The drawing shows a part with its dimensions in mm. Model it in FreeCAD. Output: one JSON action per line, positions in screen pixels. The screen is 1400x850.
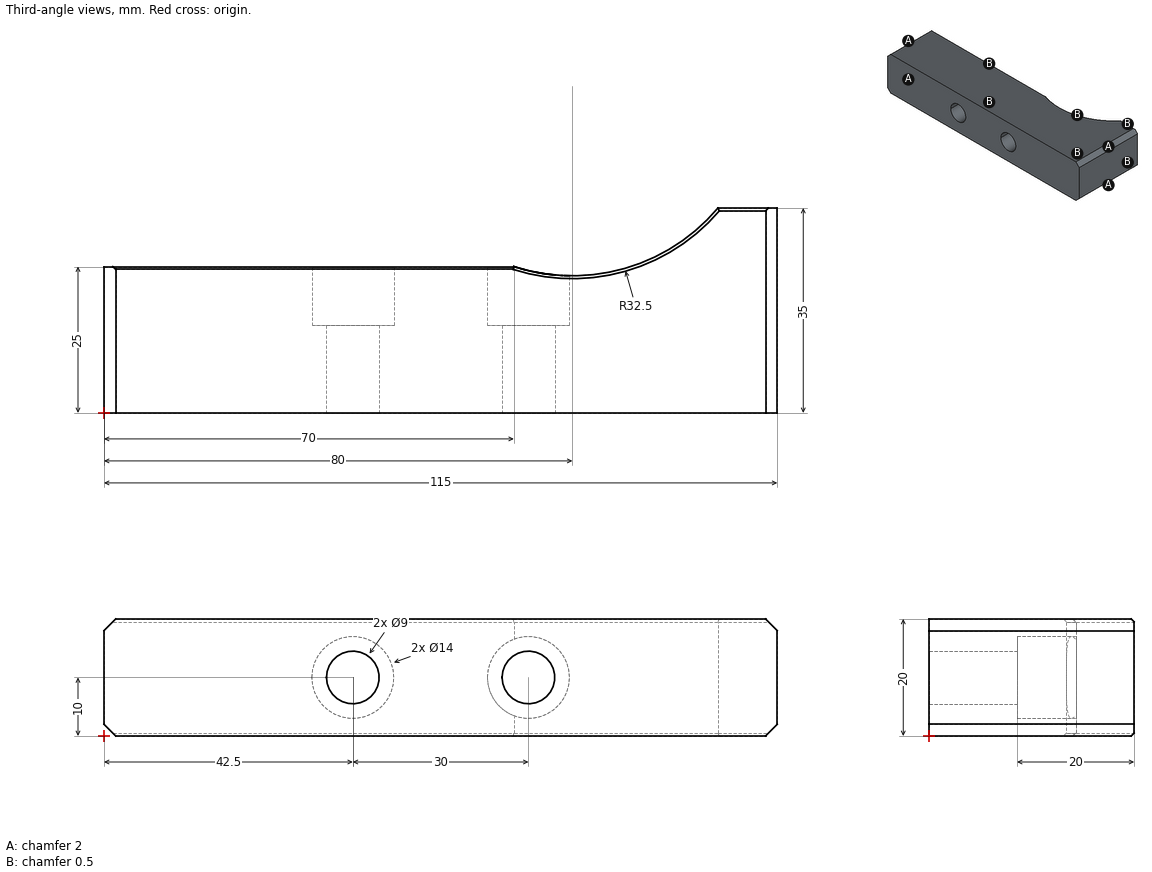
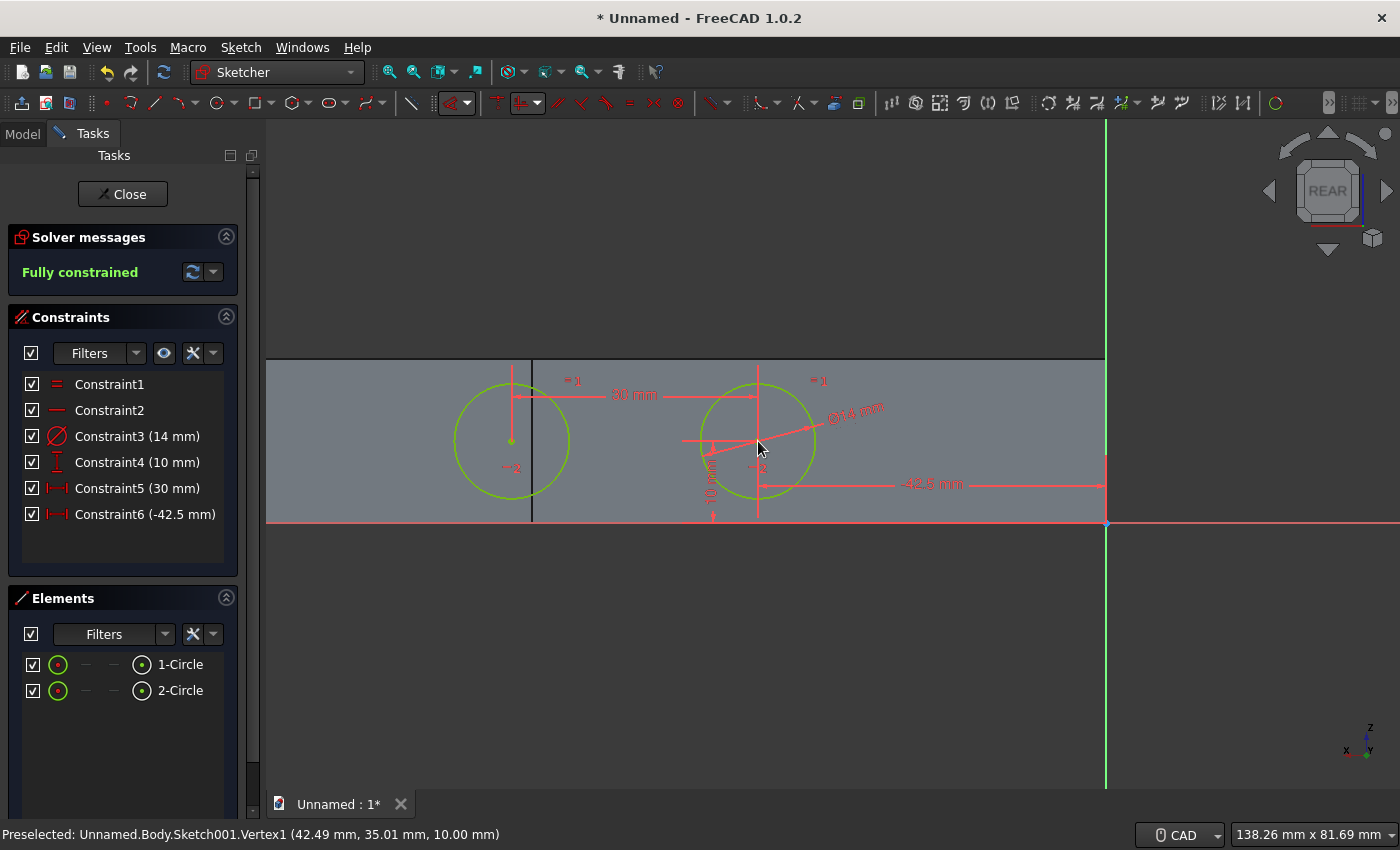
{"action": "left_click", "coordinate": [123, 194]}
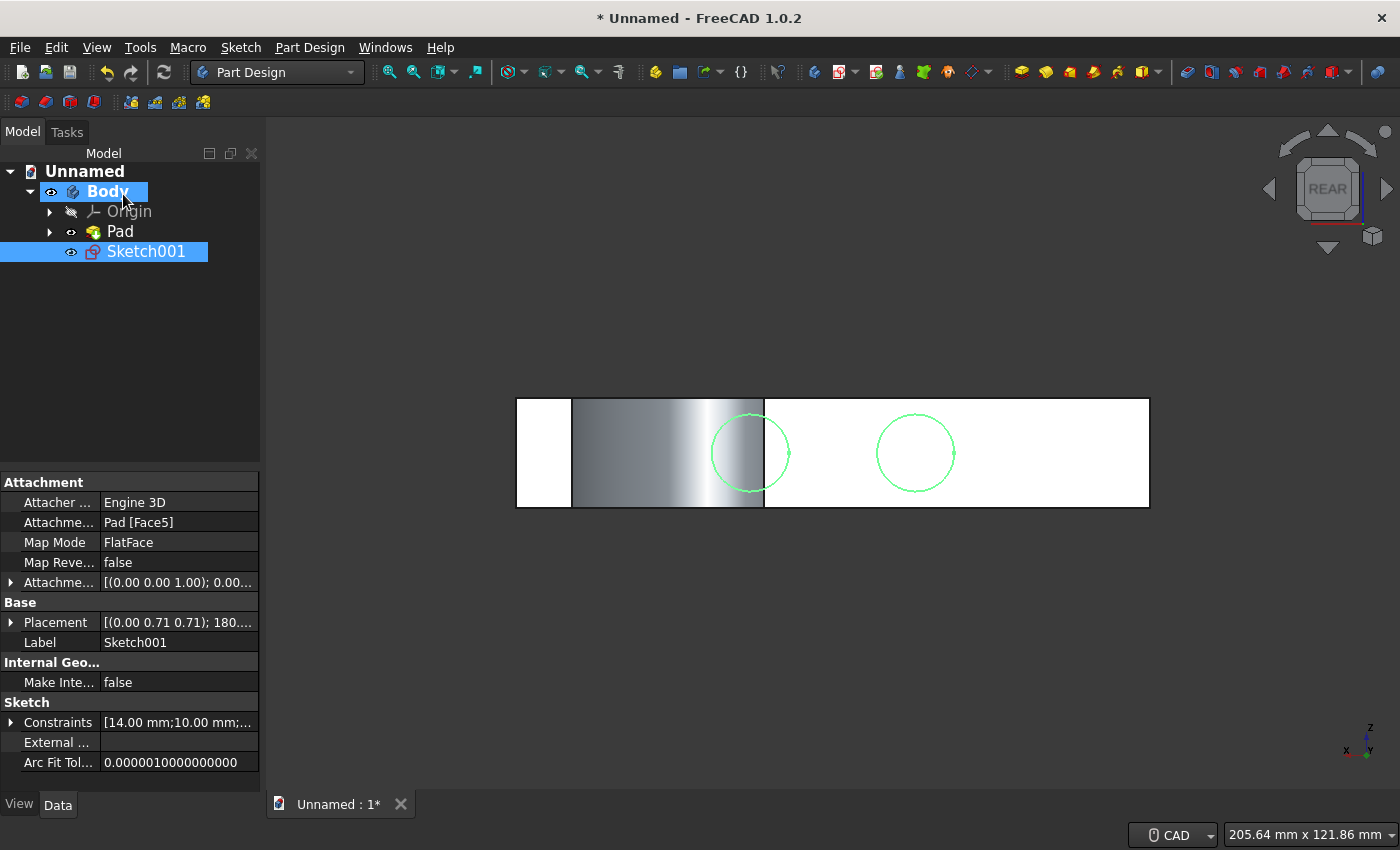
{"action": "left_click", "coordinate": [1188, 72]}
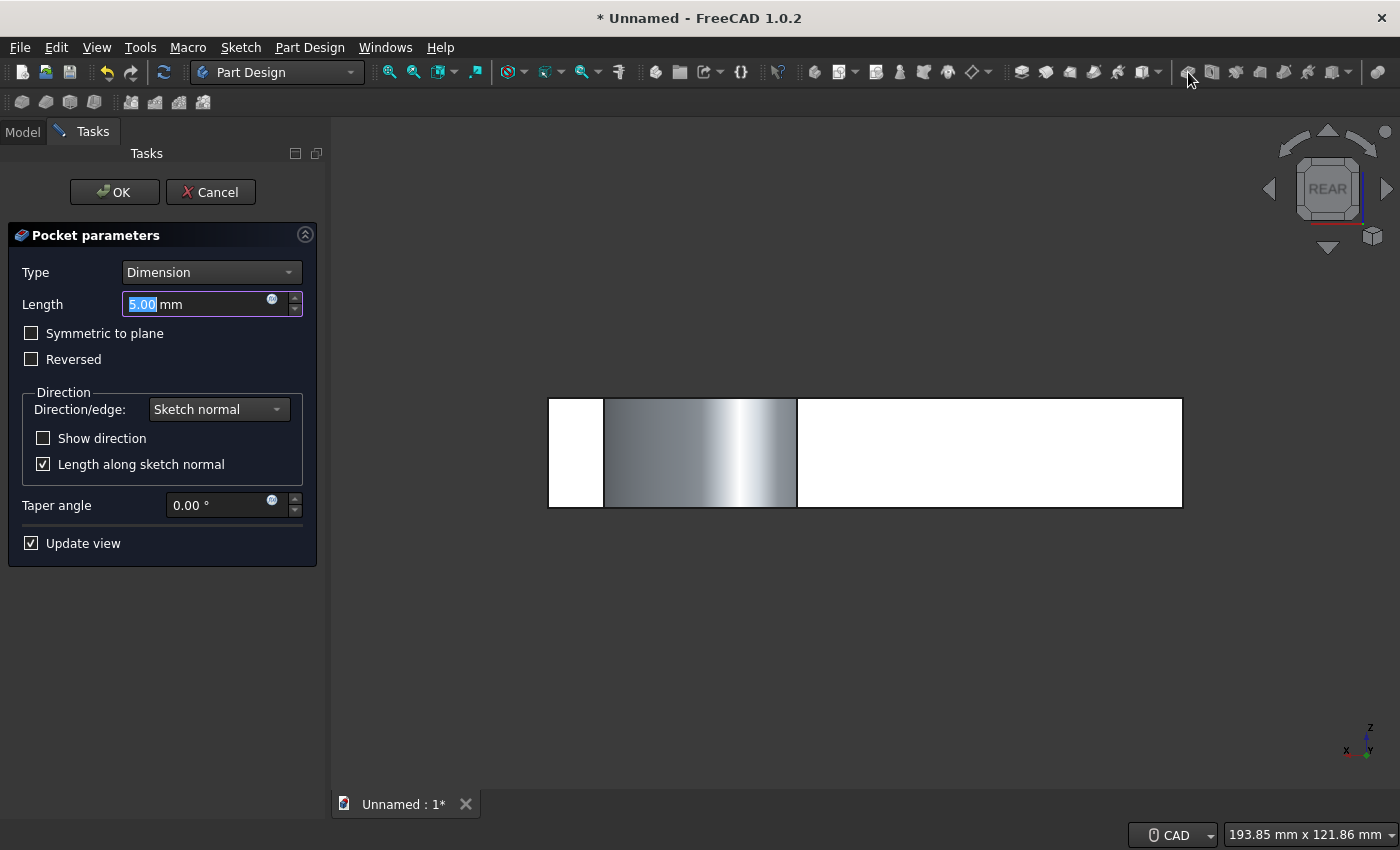
{"action": "type", "text": "20"}
{"action": "key", "text": "Tab"}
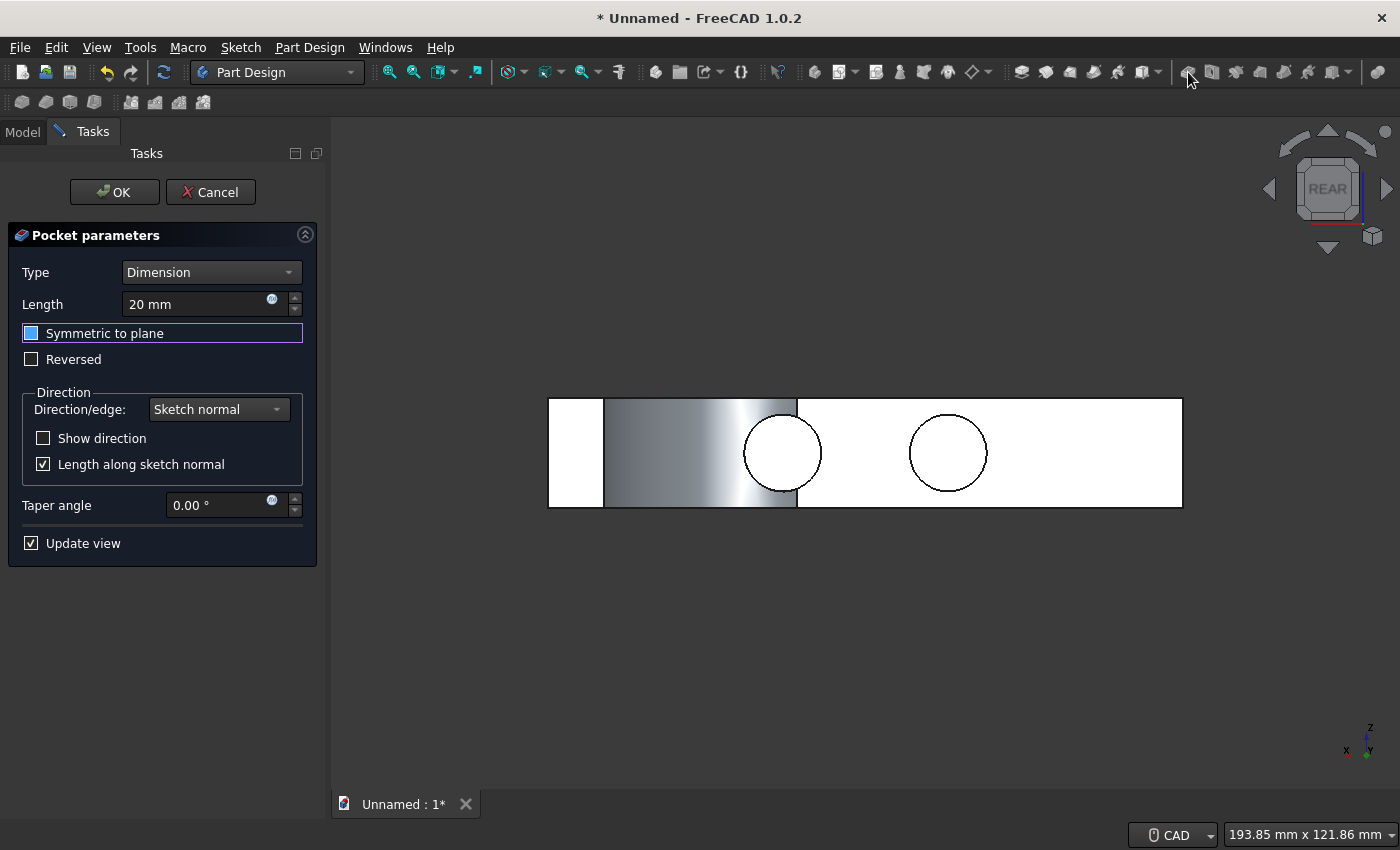
{"action": "left_click", "coordinate": [115, 192]}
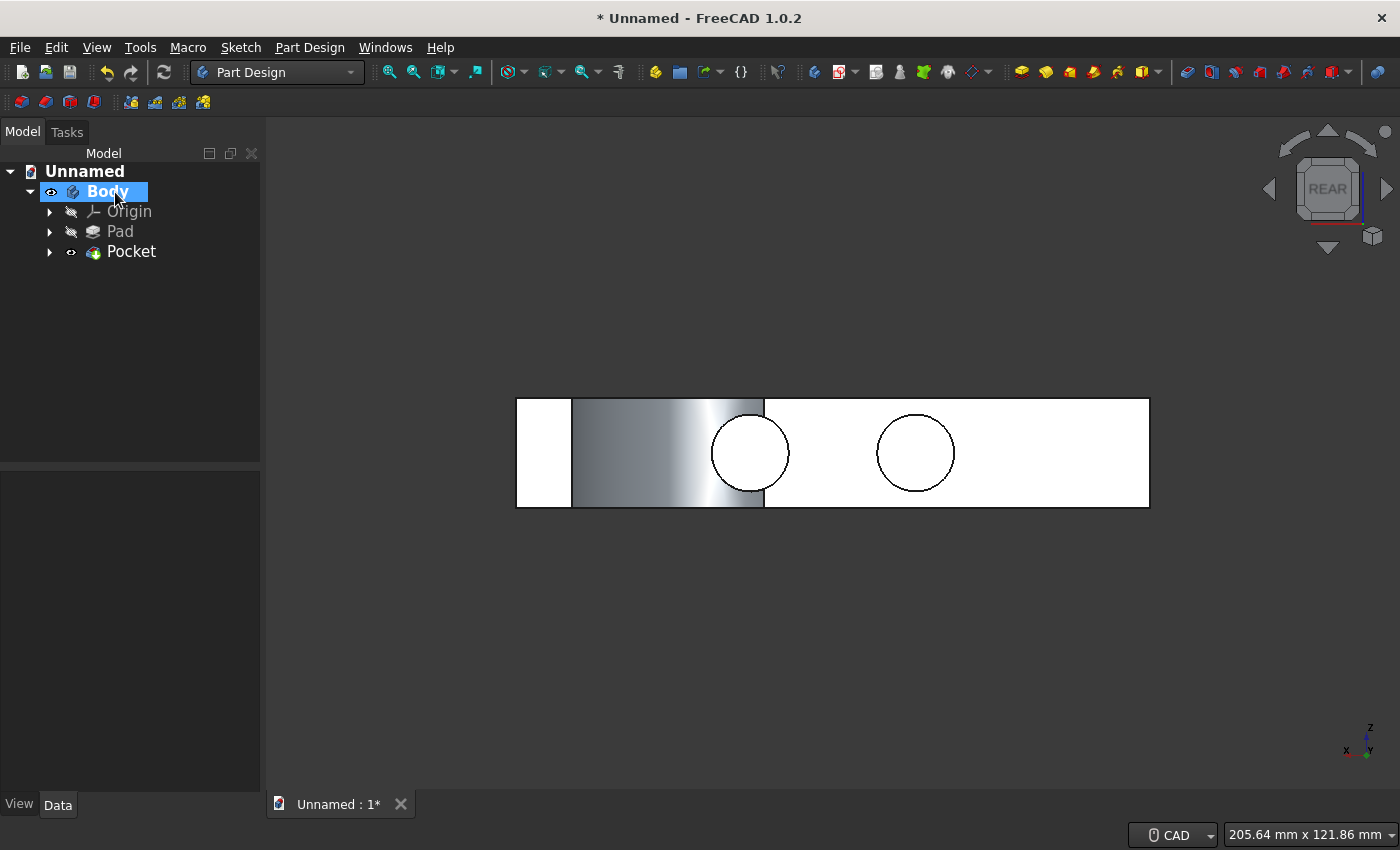
{"action": "left_click", "coordinate": [916, 452]}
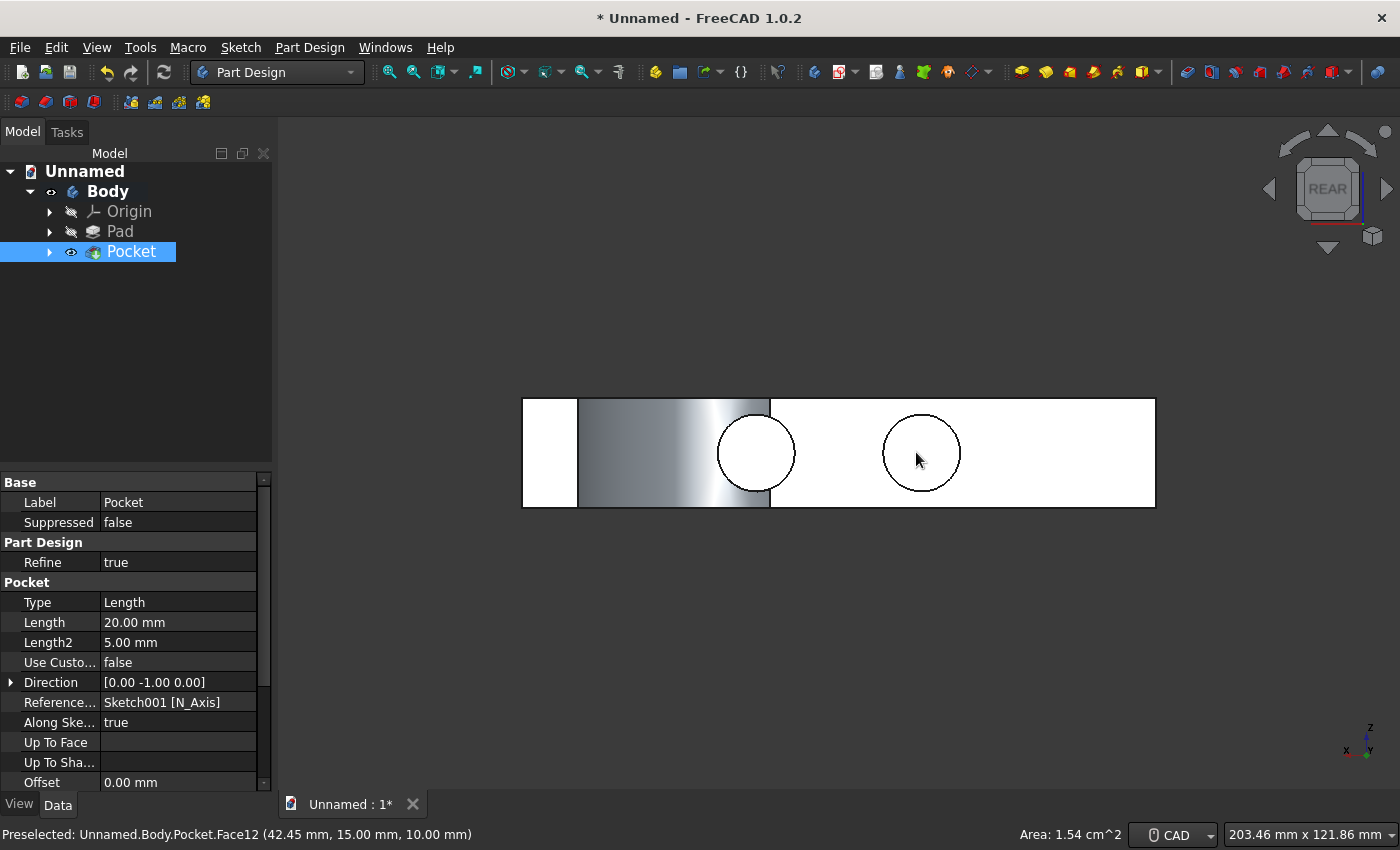
{"action": "left_click", "coordinate": [840, 72]}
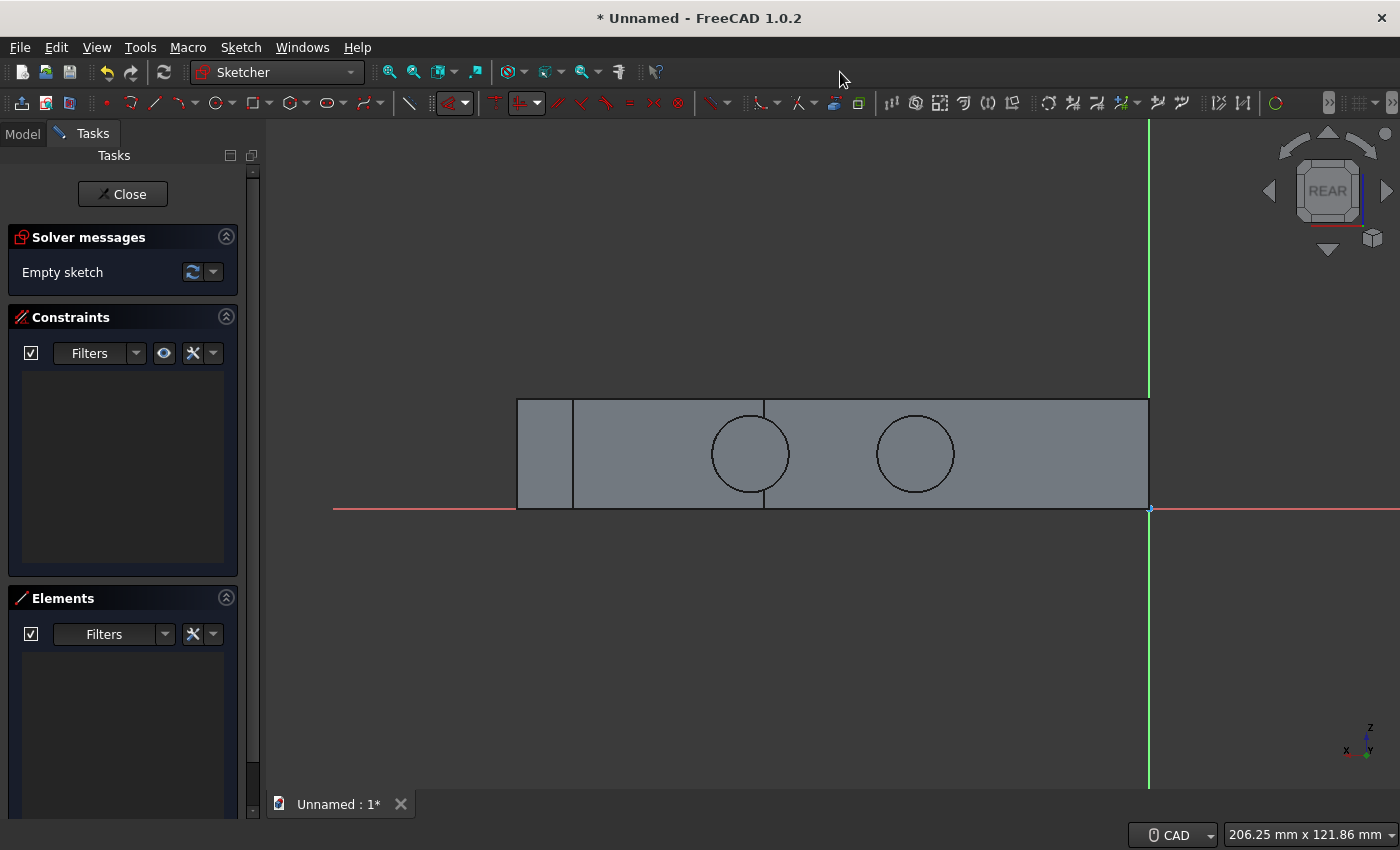
{"action": "left_click", "coordinate": [70, 104]}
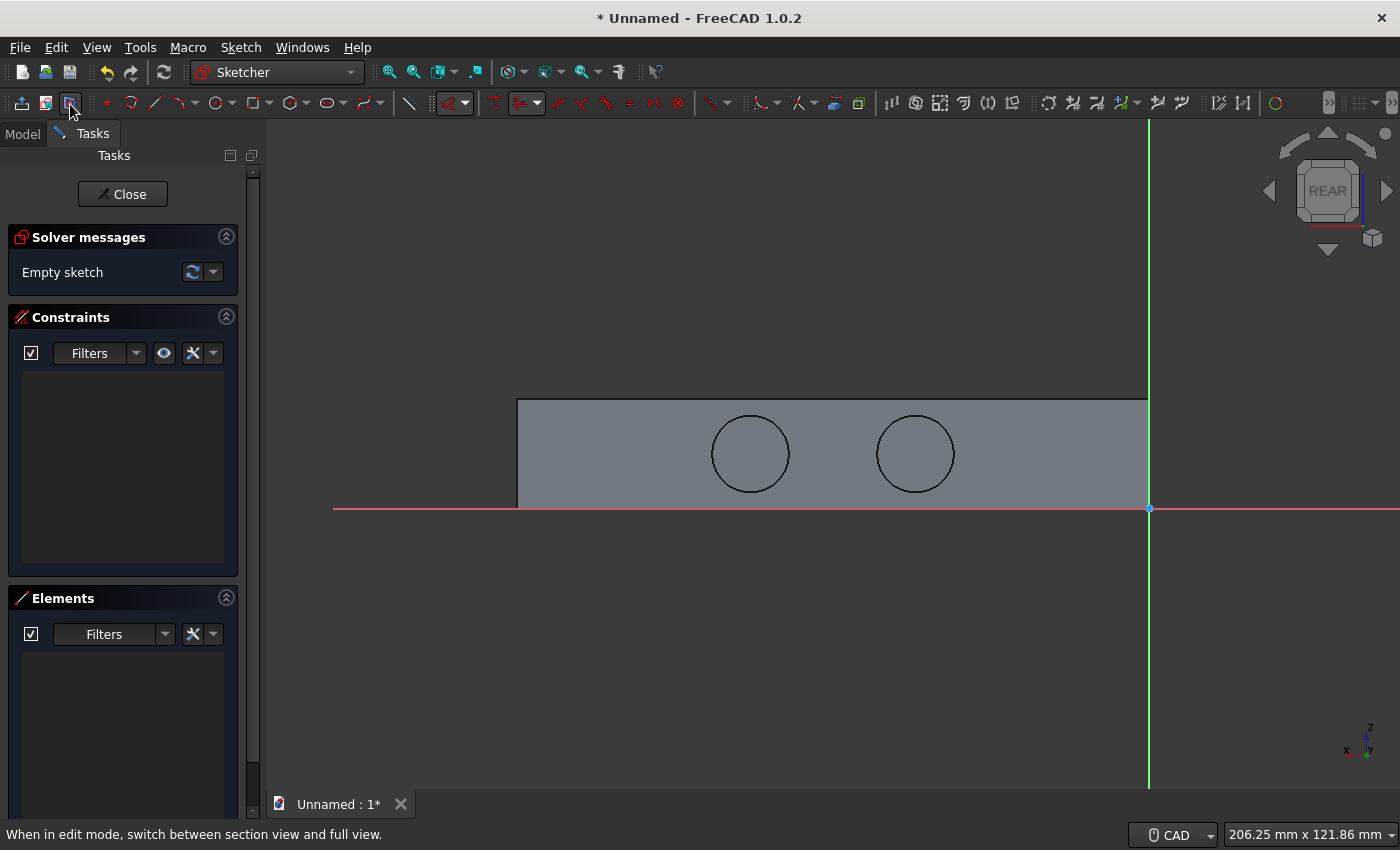
{"action": "scroll", "coordinate": [1235, 500], "scroll_direction": "up", "scroll_amount": 2}